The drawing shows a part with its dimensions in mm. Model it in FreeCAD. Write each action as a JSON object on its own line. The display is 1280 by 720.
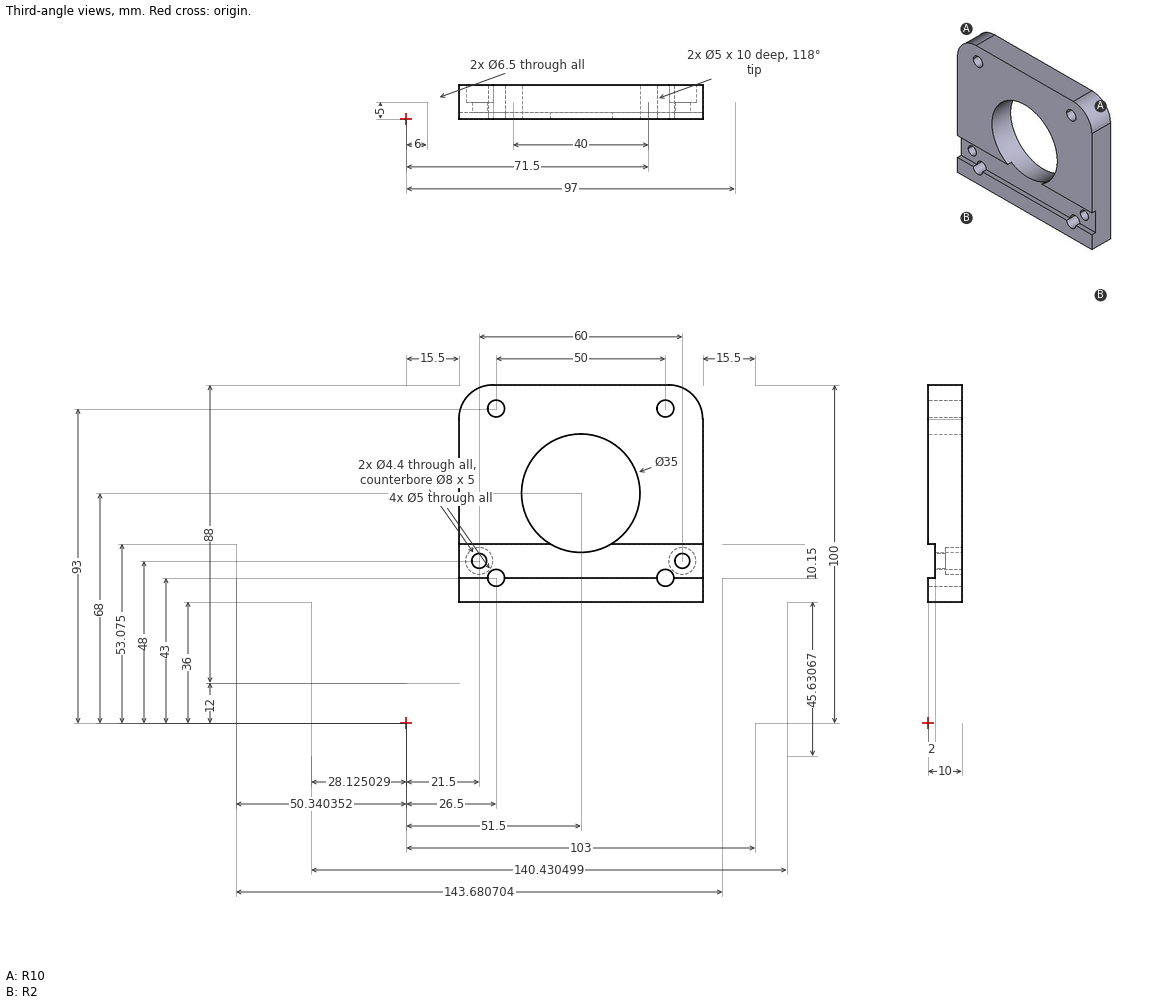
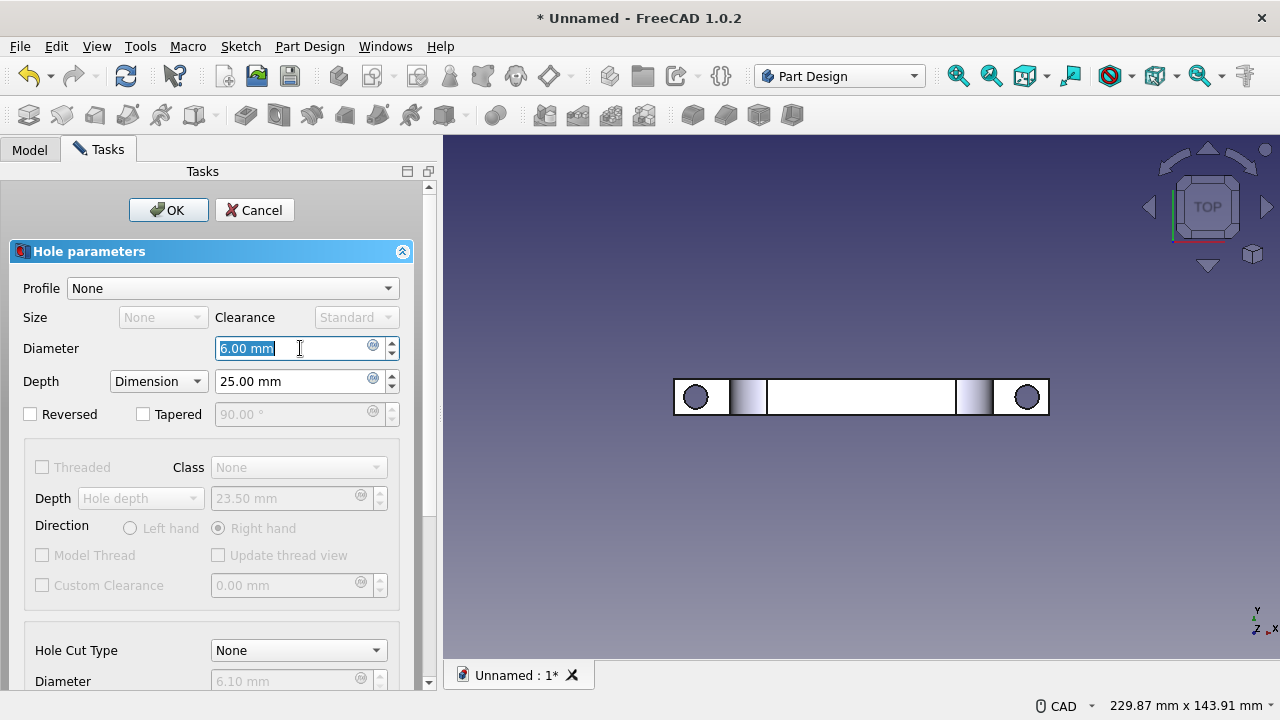
{"action": "type", "text": "5"}
{"action": "key", "text": "Tab"}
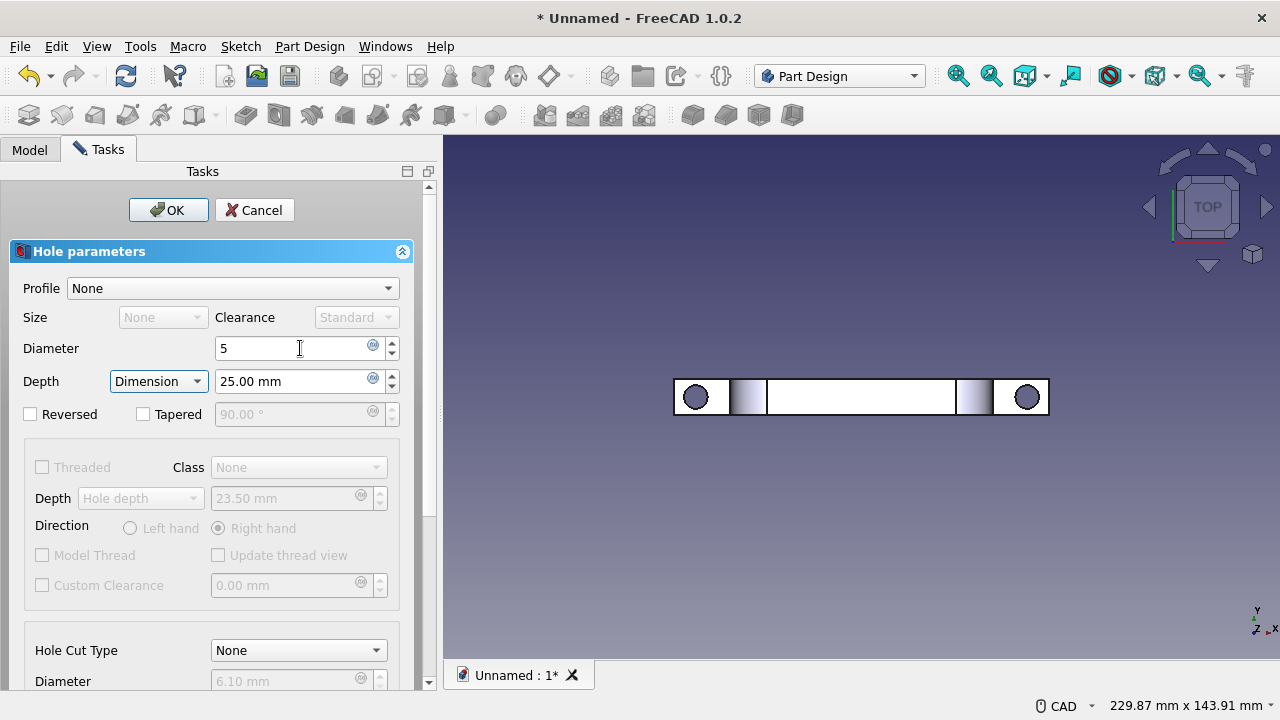
{"action": "triple_click", "coordinate": [300, 382]}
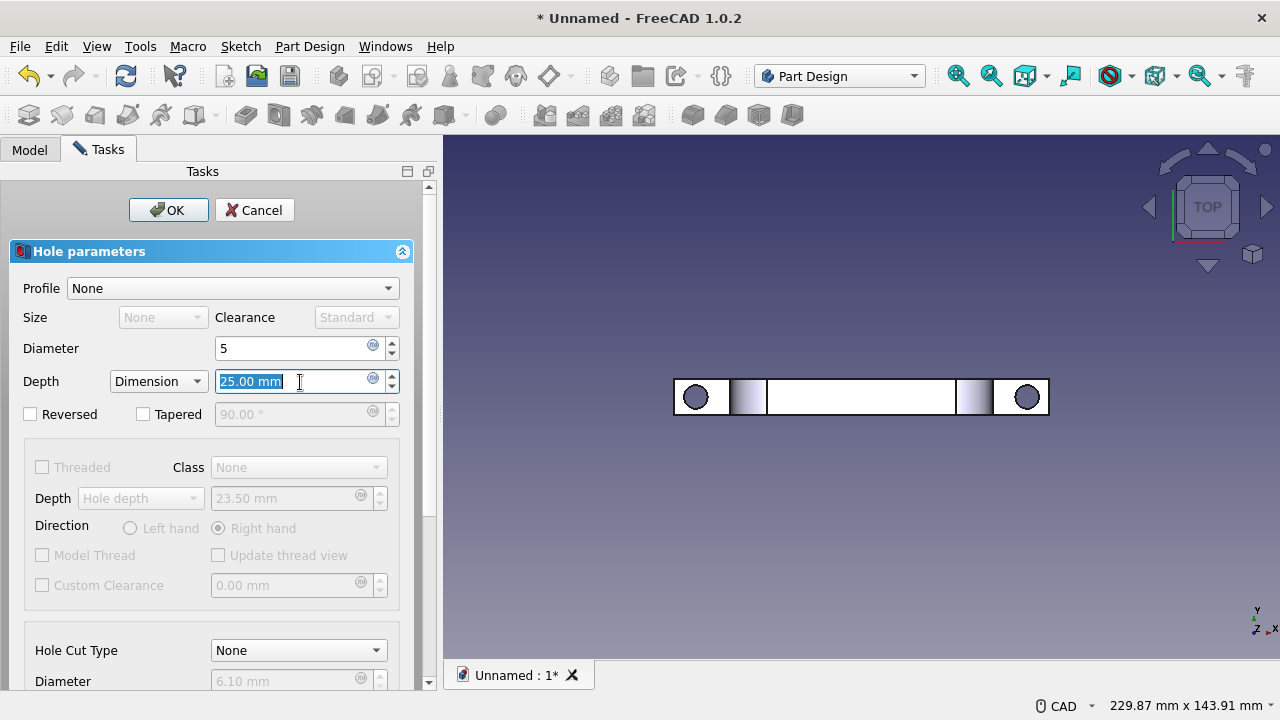
{"action": "type", "text": "10"}
{"action": "key", "text": "Tab"}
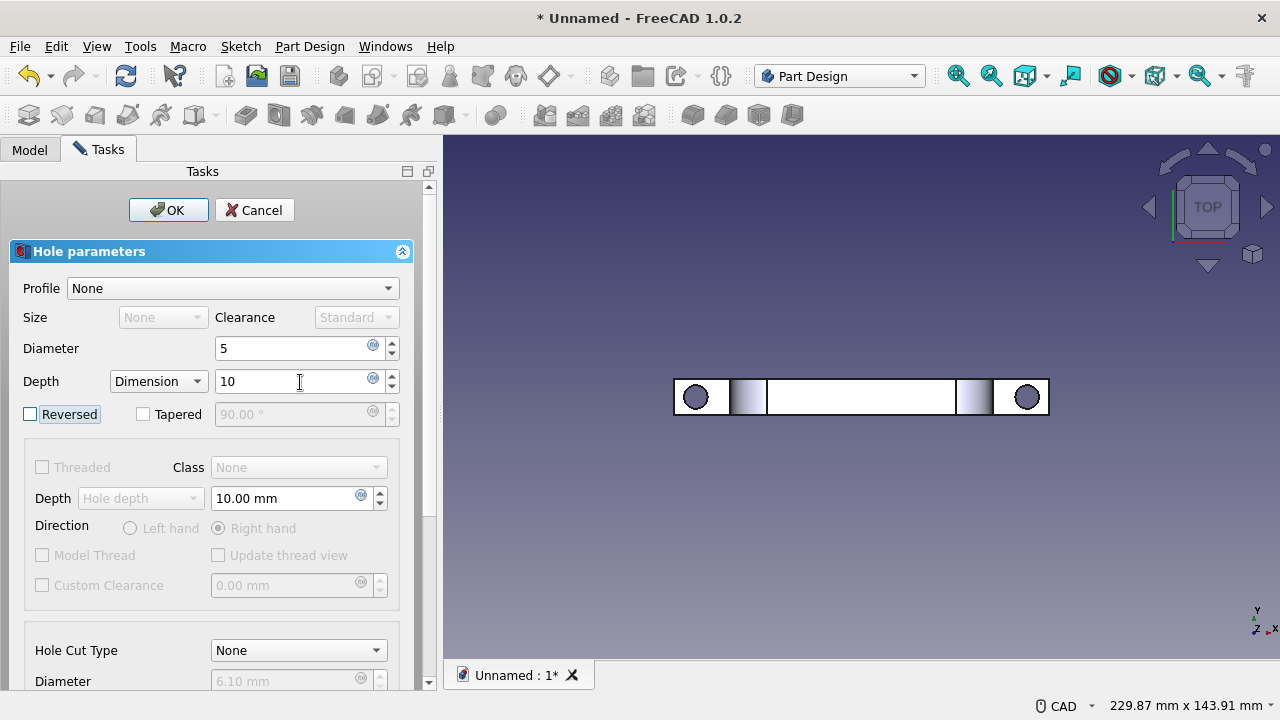
{"action": "left_click", "coordinate": [31, 414]}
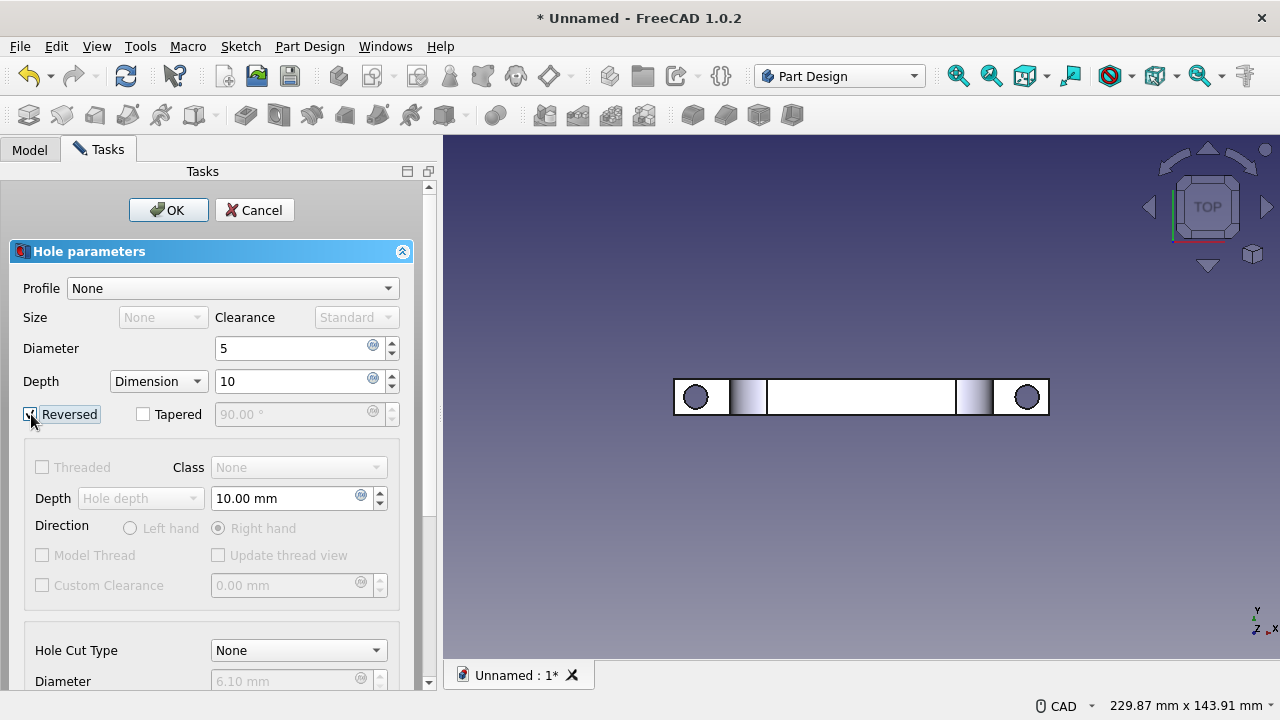
{"action": "left_click", "coordinate": [169, 210]}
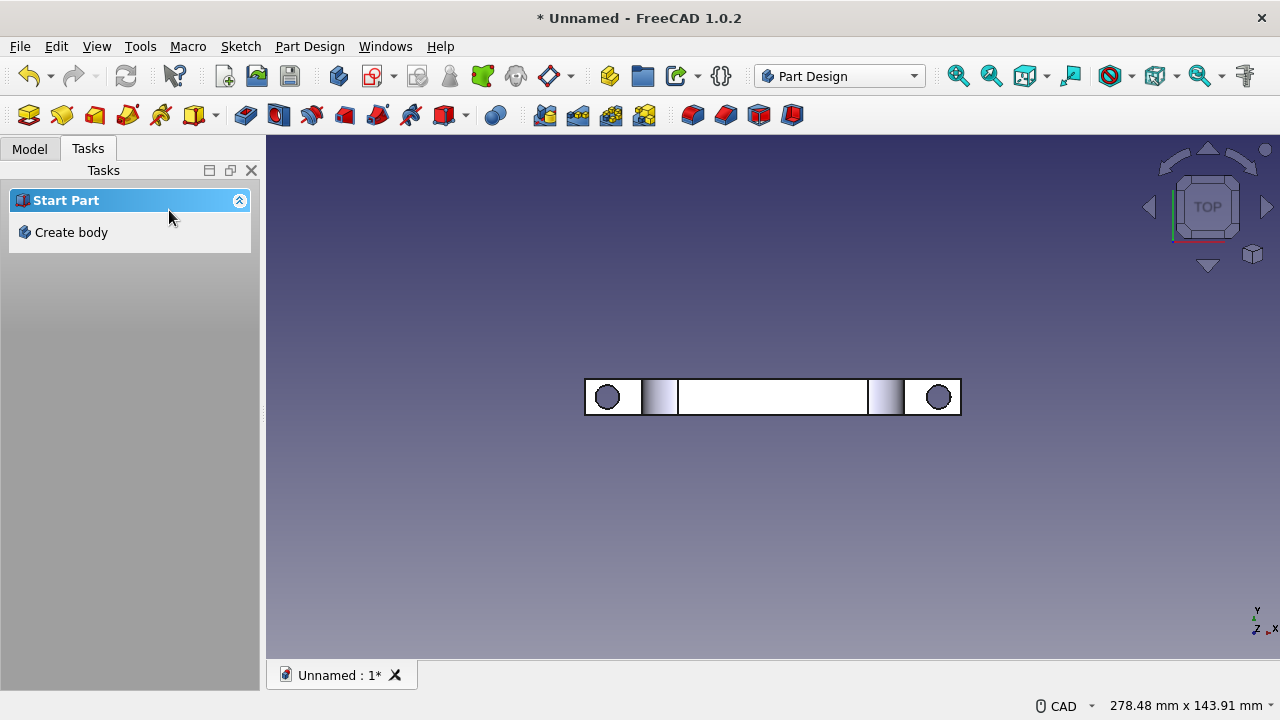
{"action": "key", "text": "v f"}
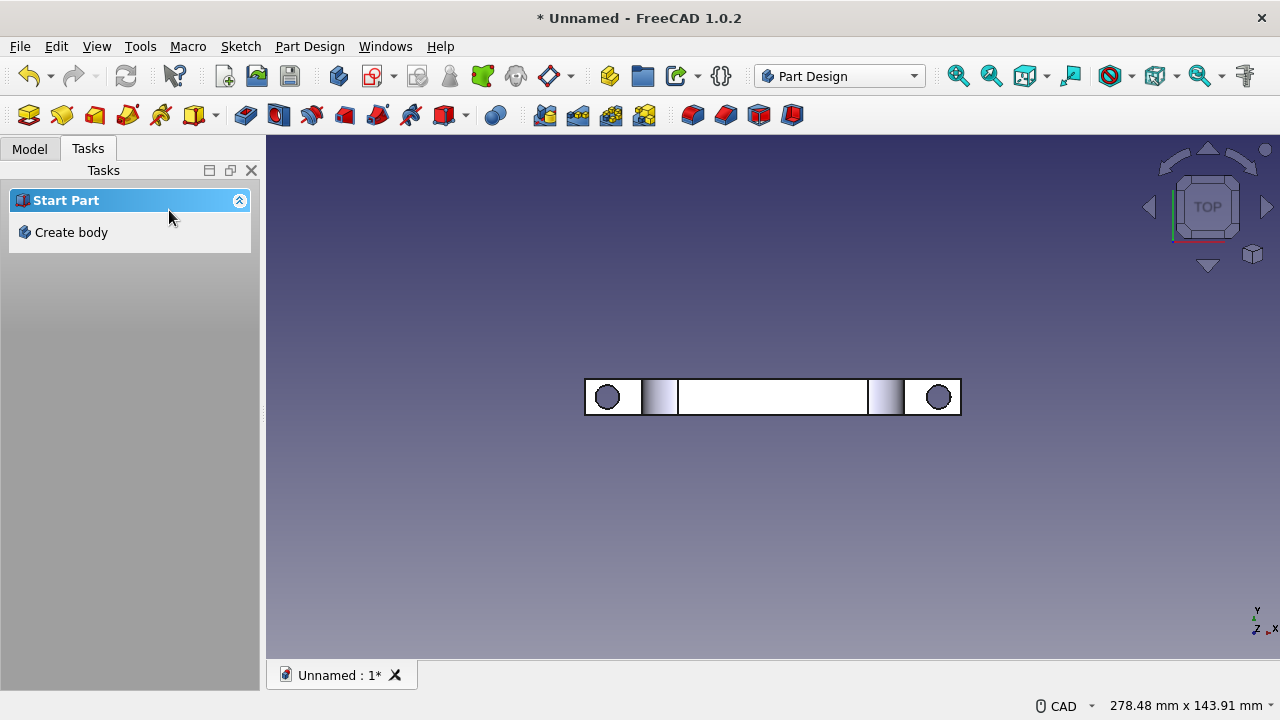
{"action": "key", "text": "0"}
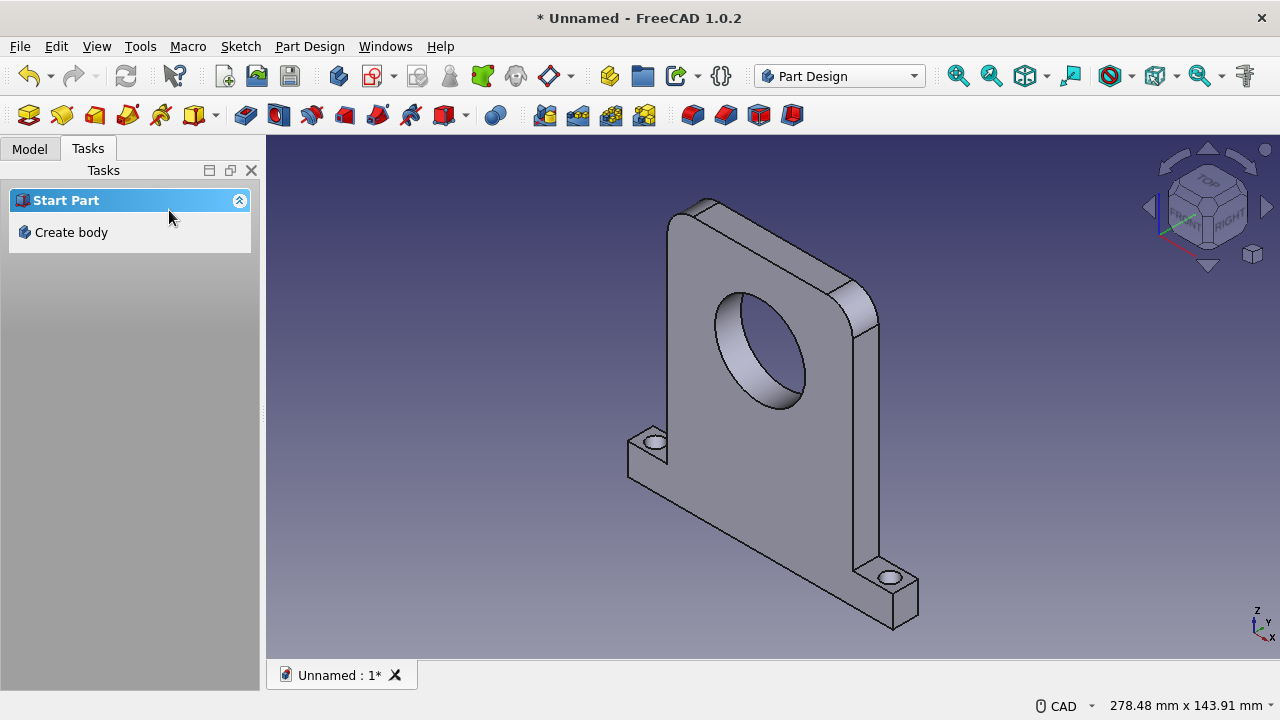
{"action": "key", "text": "2"}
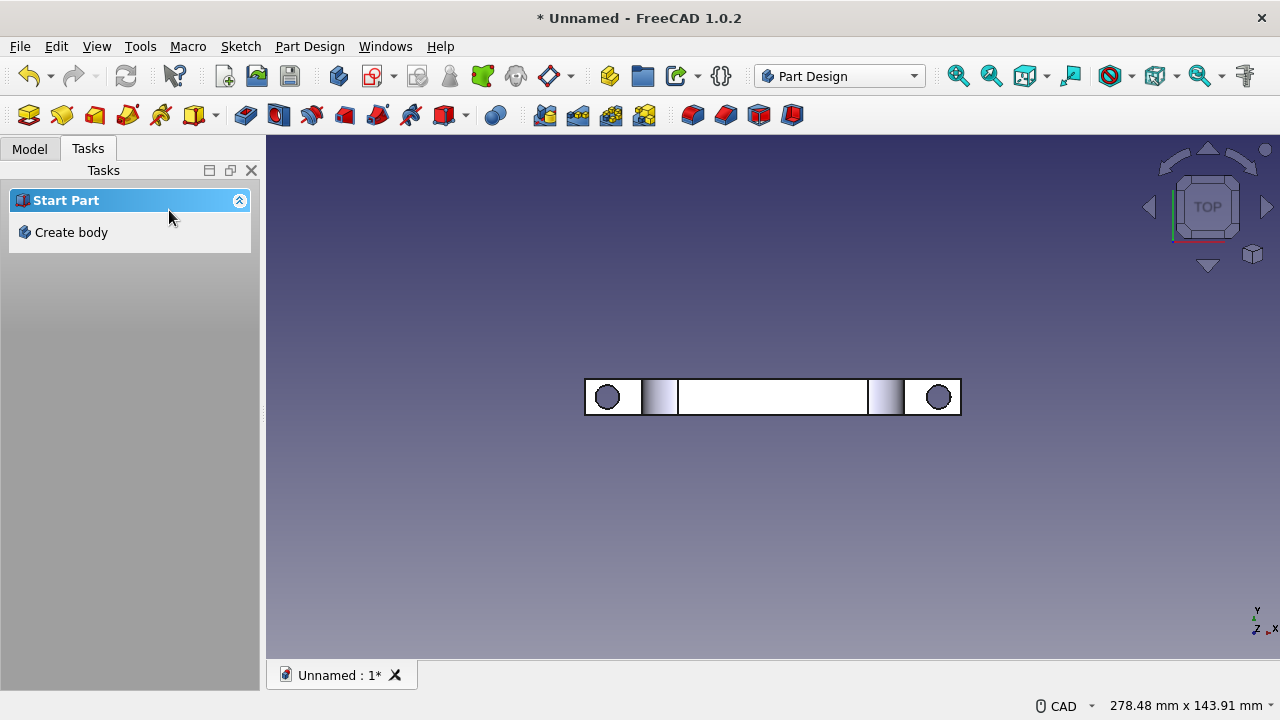
{"action": "left_click", "coordinate": [959, 76]}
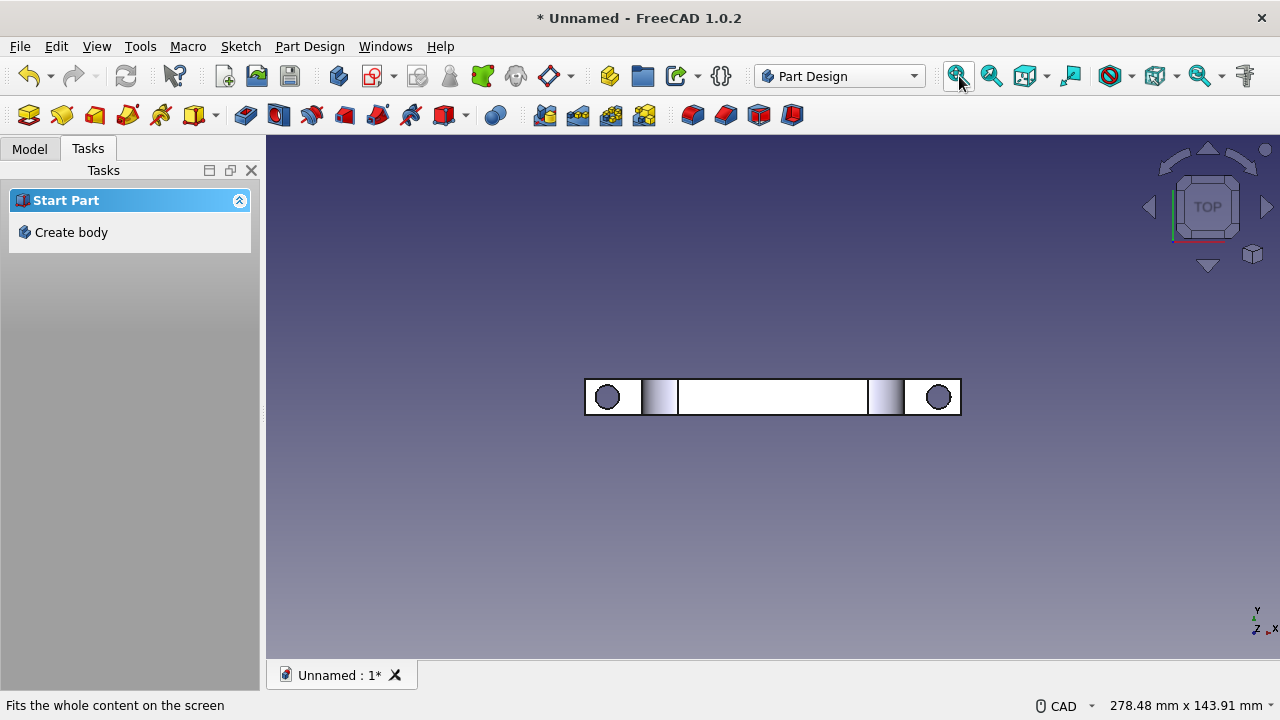
{"action": "key", "text": "1"}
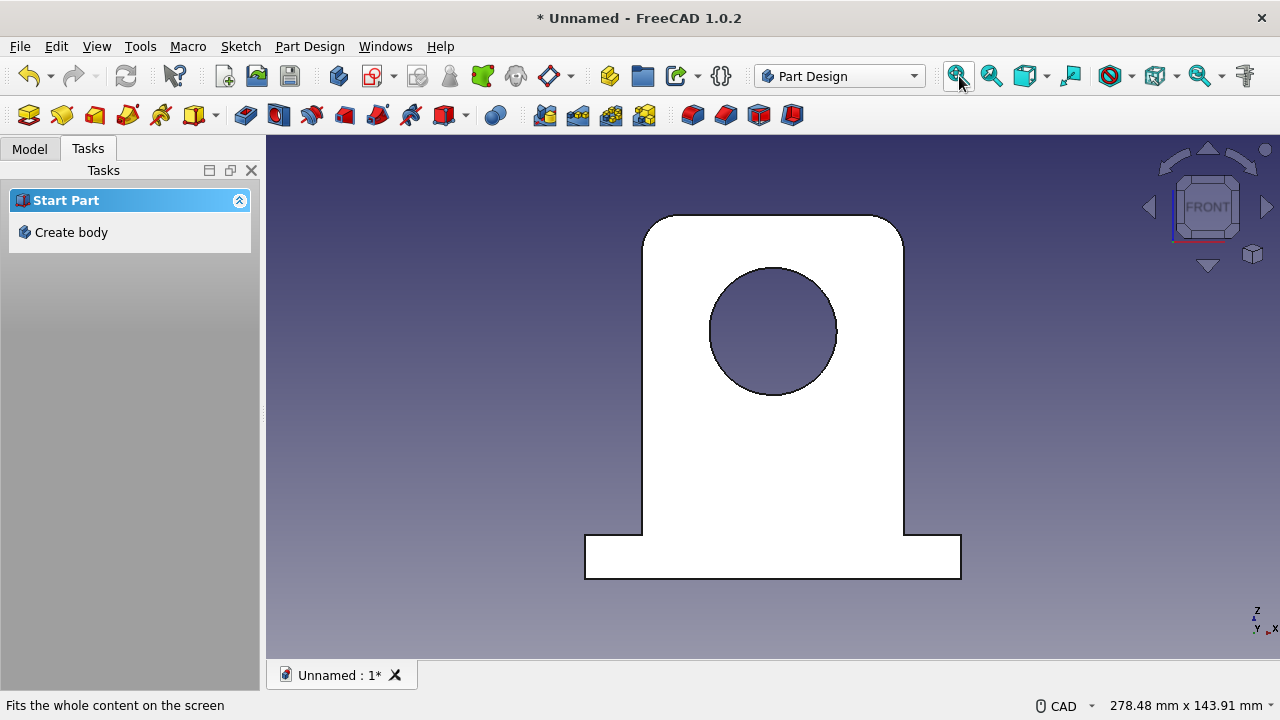
{"action": "key", "text": "3"}